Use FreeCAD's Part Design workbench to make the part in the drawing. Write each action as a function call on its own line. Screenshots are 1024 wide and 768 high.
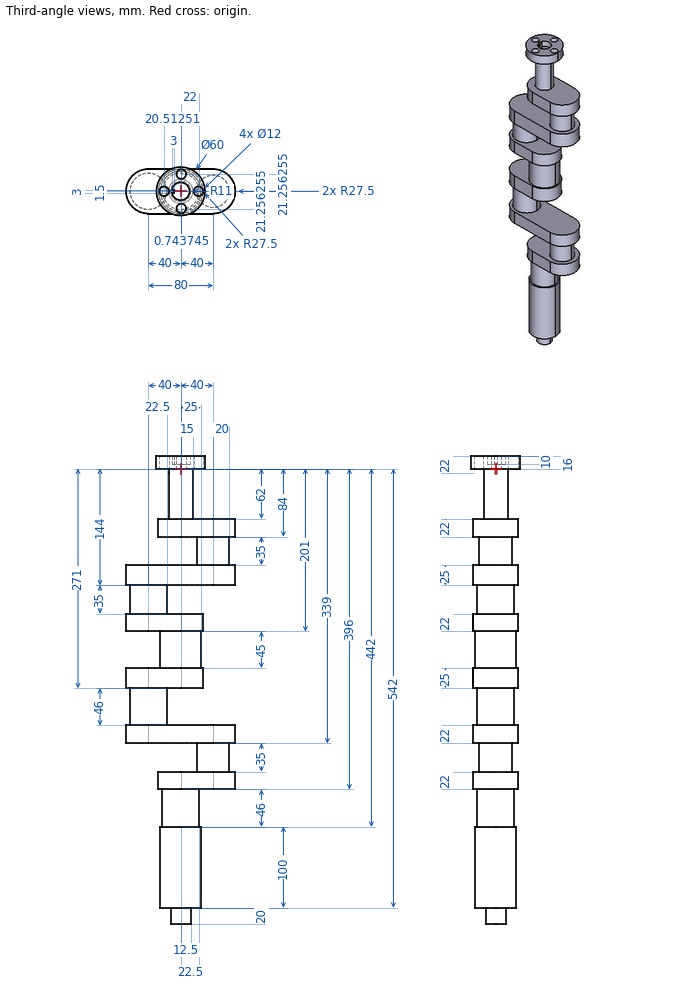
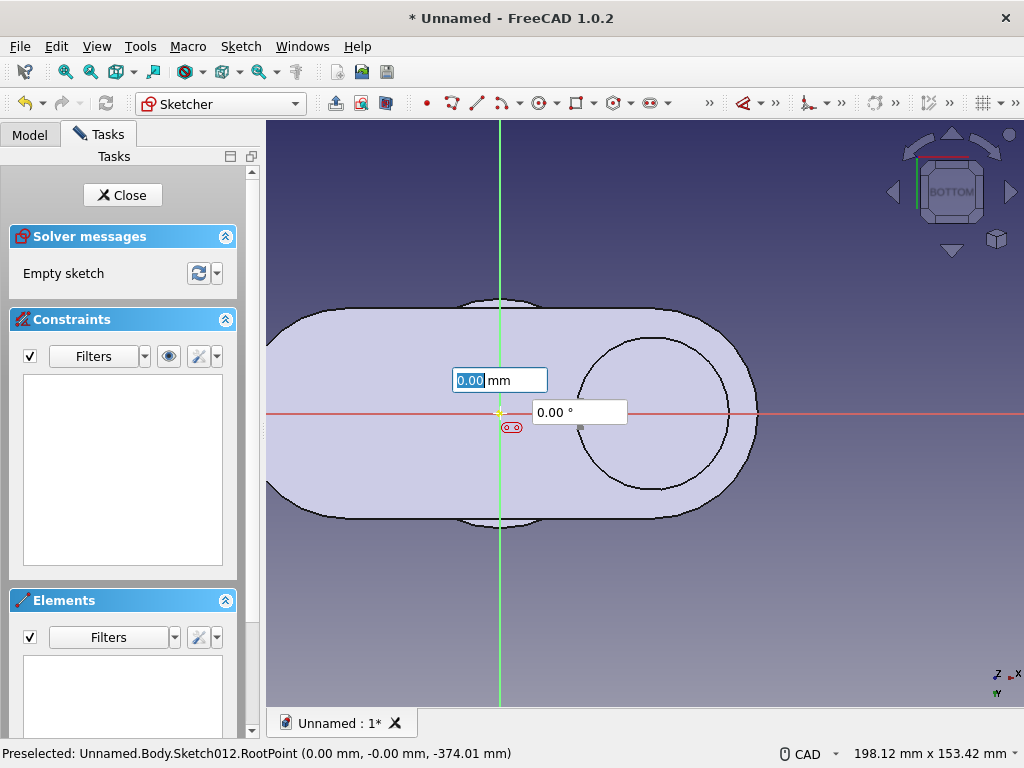
click(653, 404)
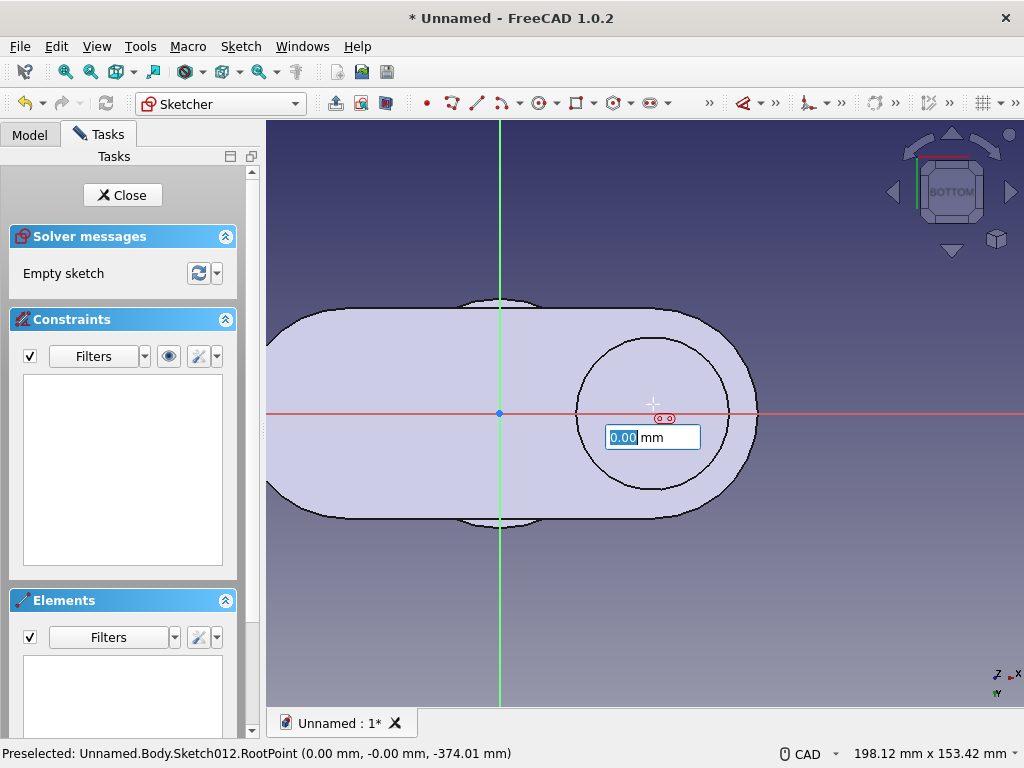
click(576, 308)
key(Escape)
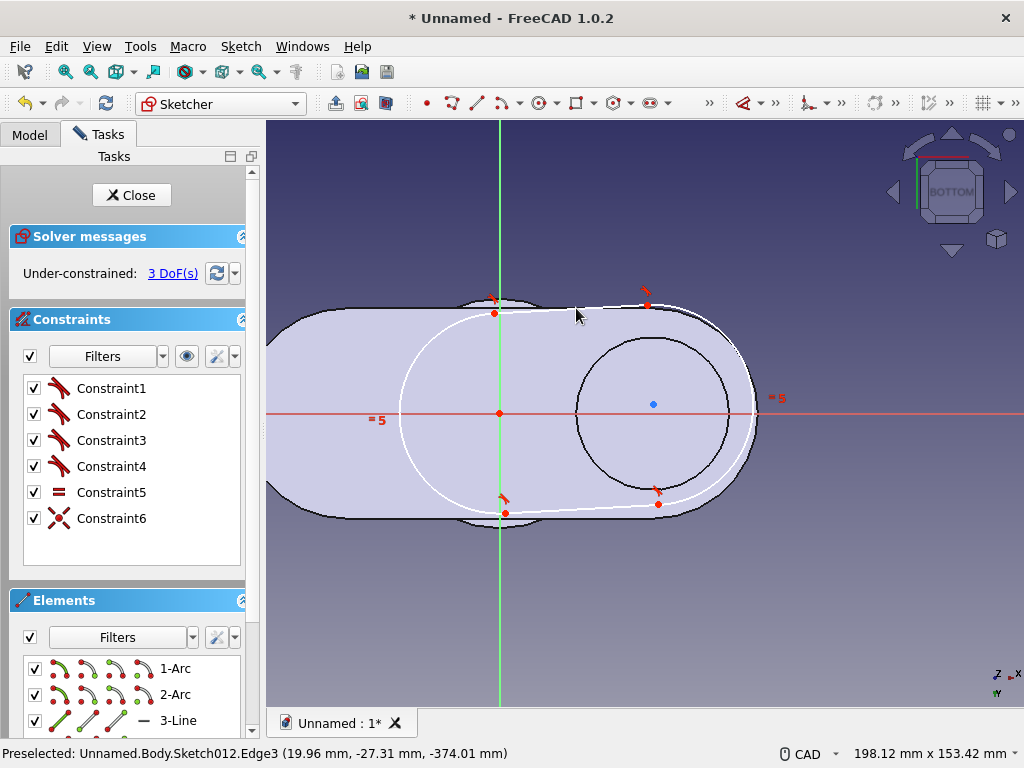
click(540, 311)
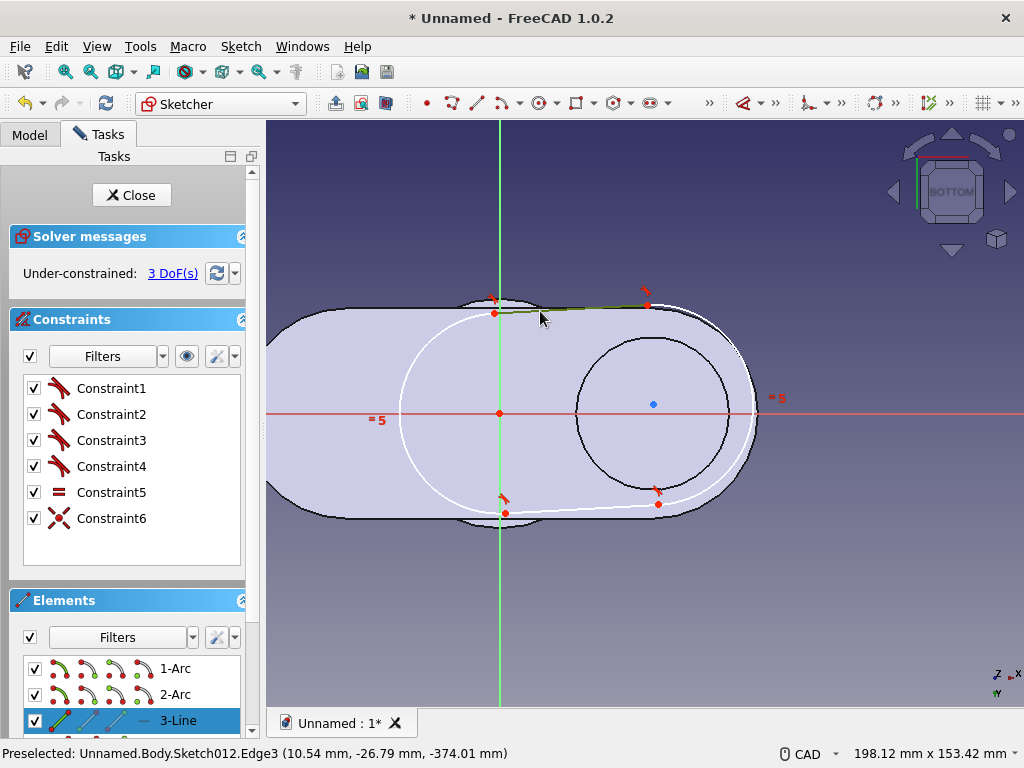
key(h)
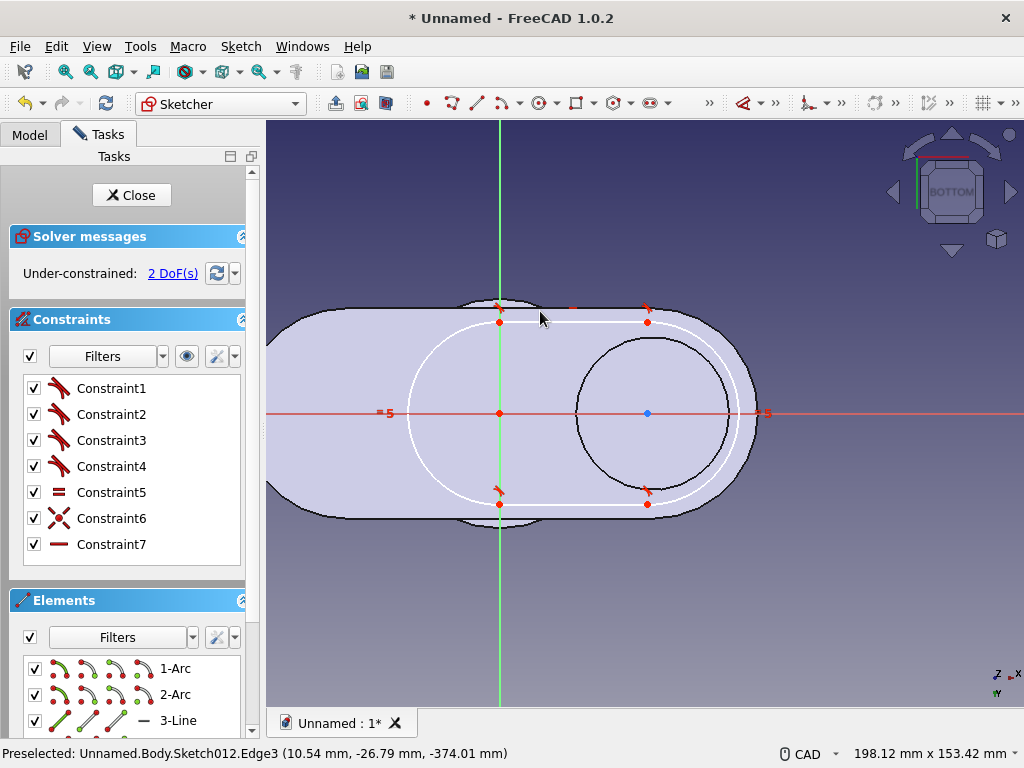
key(d)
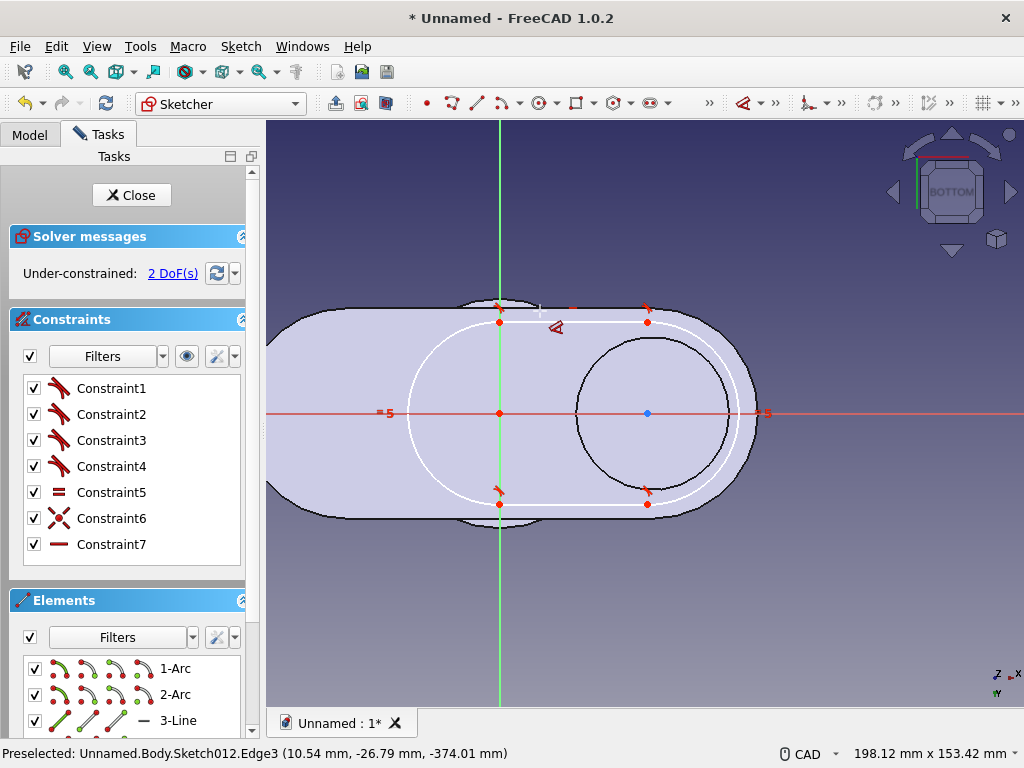
click(426, 360)
click(400, 341)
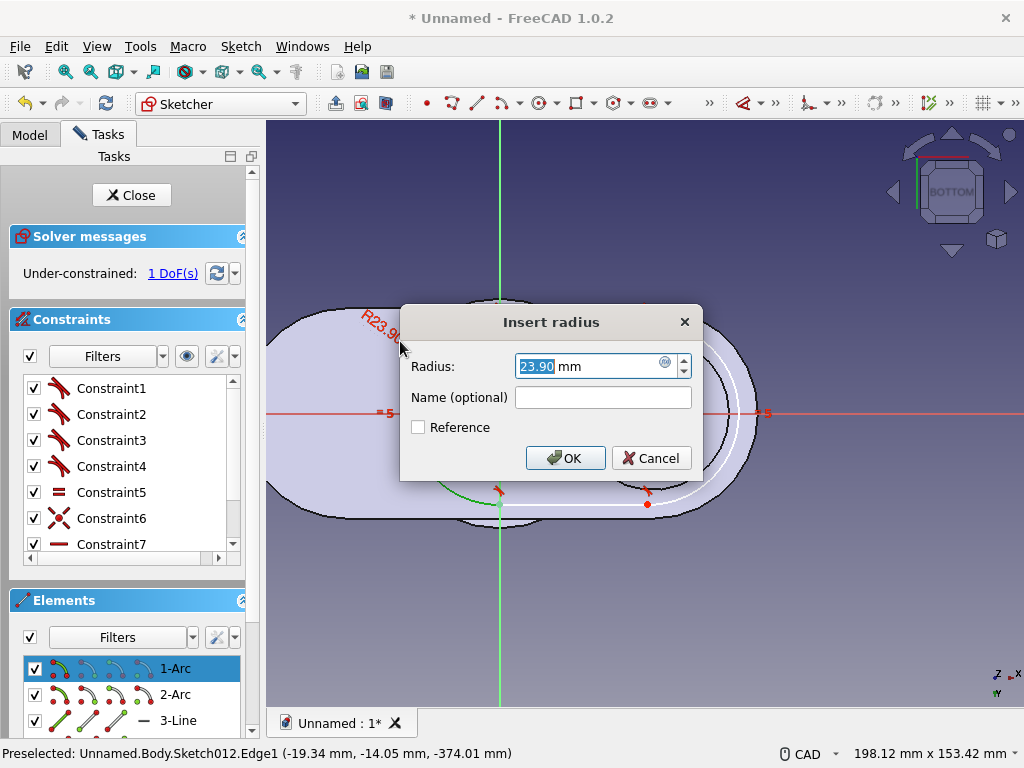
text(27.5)
key(Return)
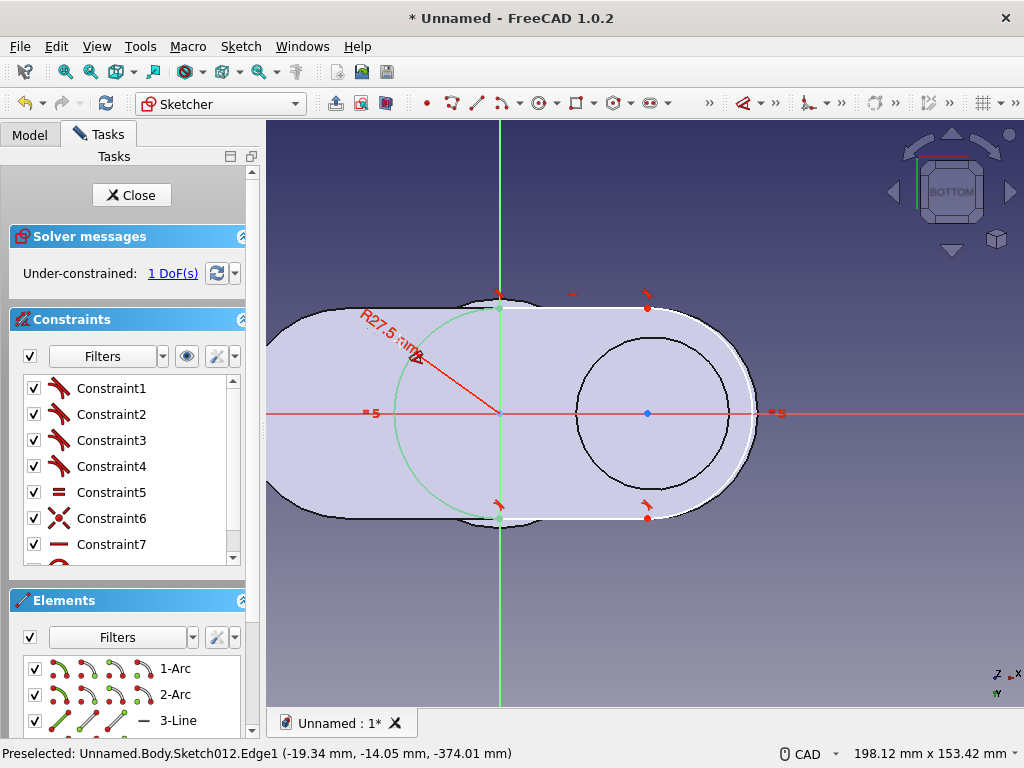
click(544, 308)
click(573, 274)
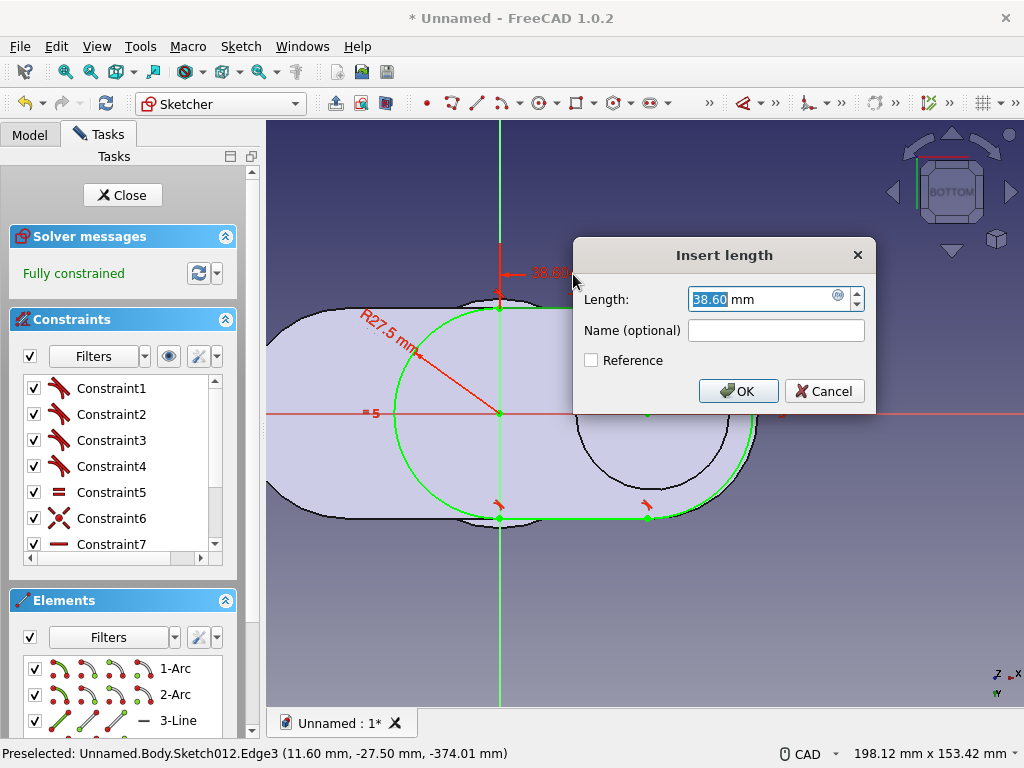
text(40)
key(Return)
key(Escape)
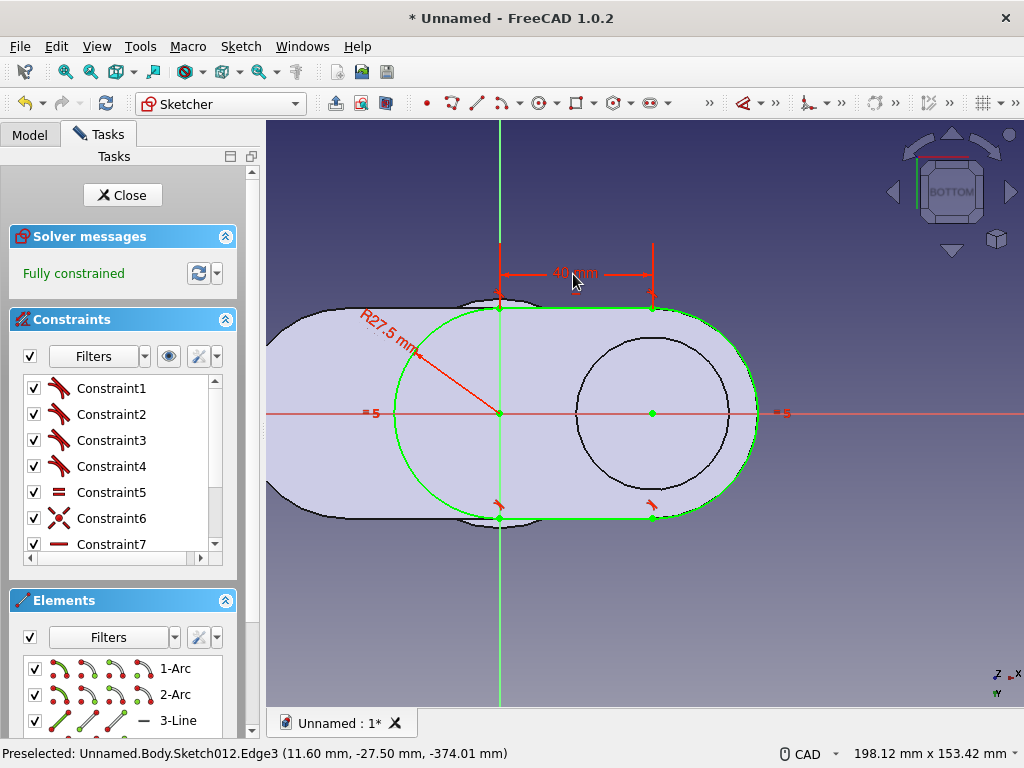
click(123, 195)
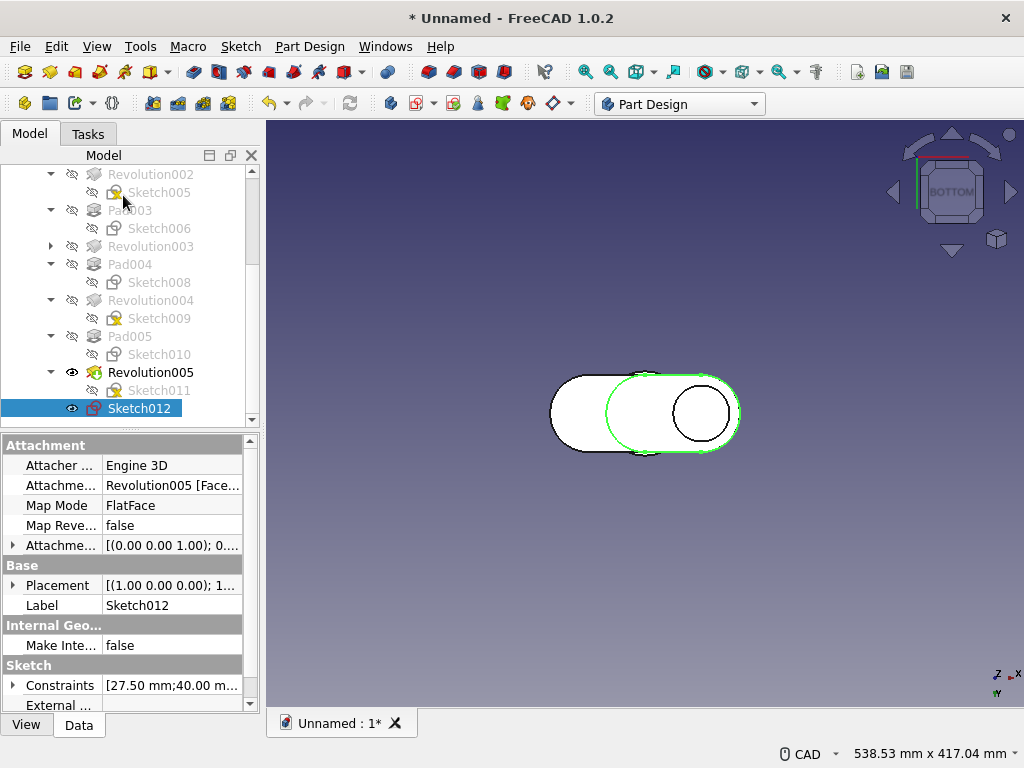
click(25, 72)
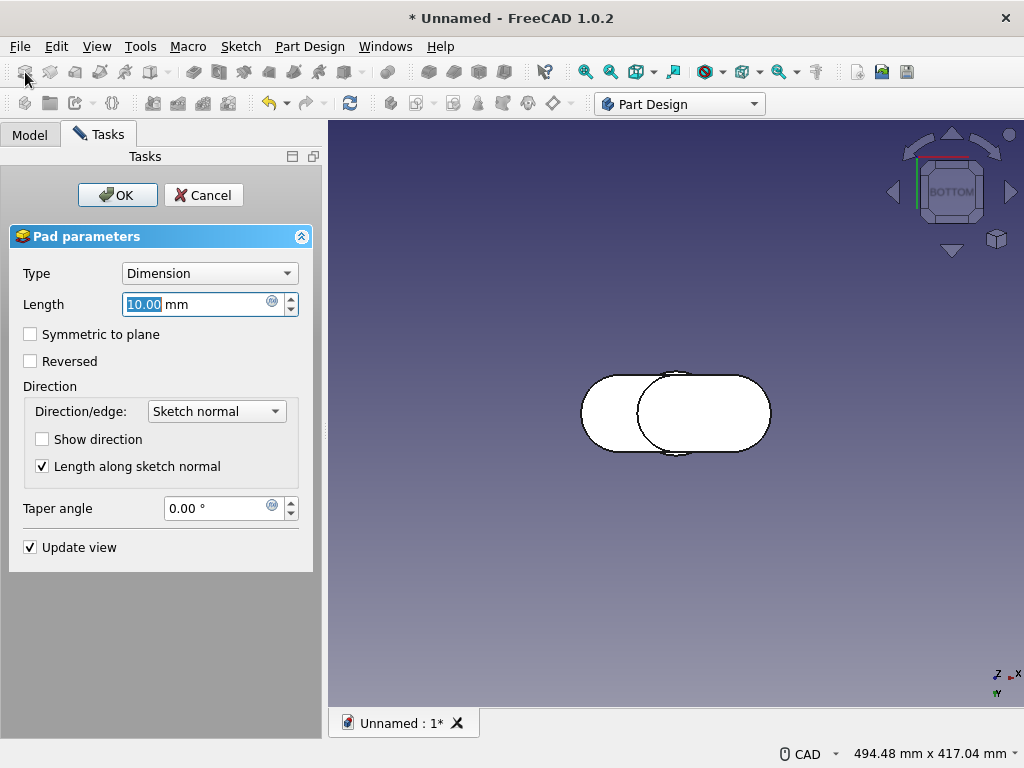
text(22)
key(Tab)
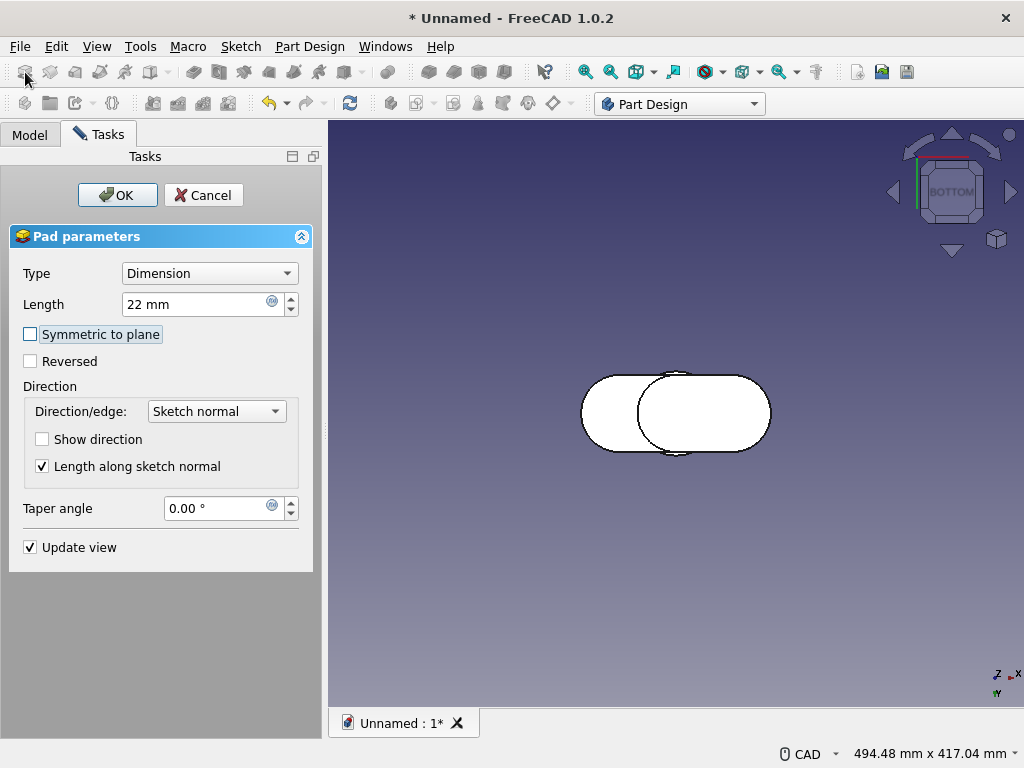
click(118, 195)